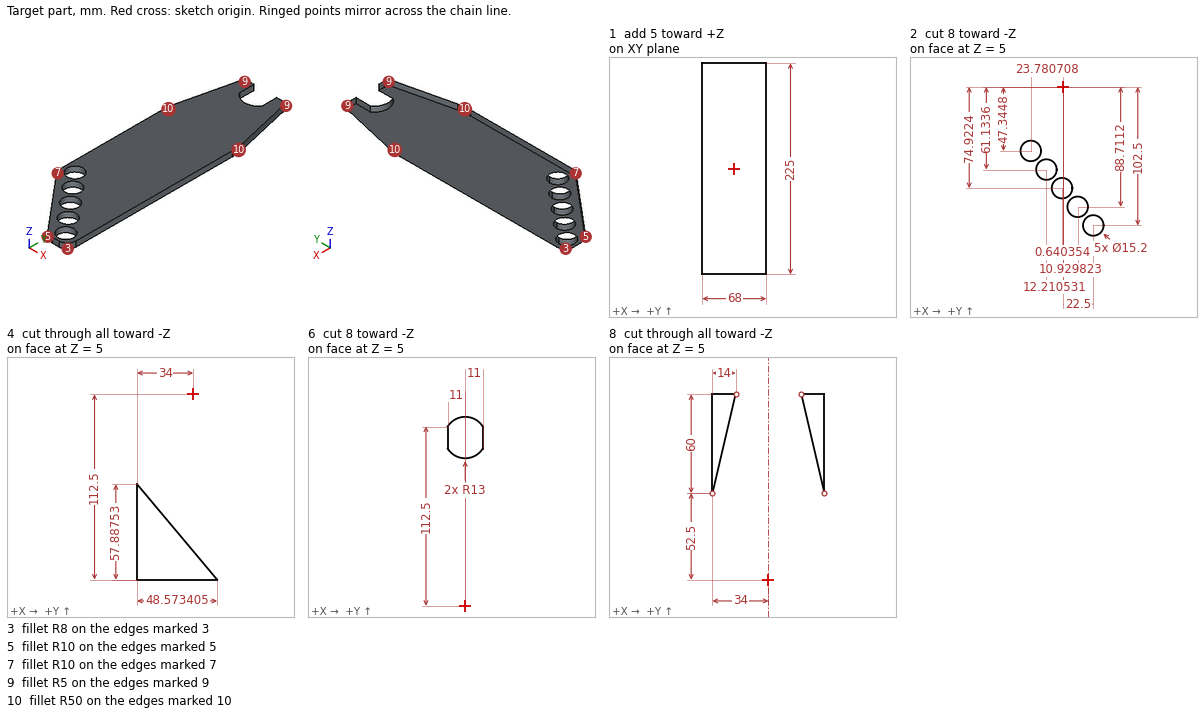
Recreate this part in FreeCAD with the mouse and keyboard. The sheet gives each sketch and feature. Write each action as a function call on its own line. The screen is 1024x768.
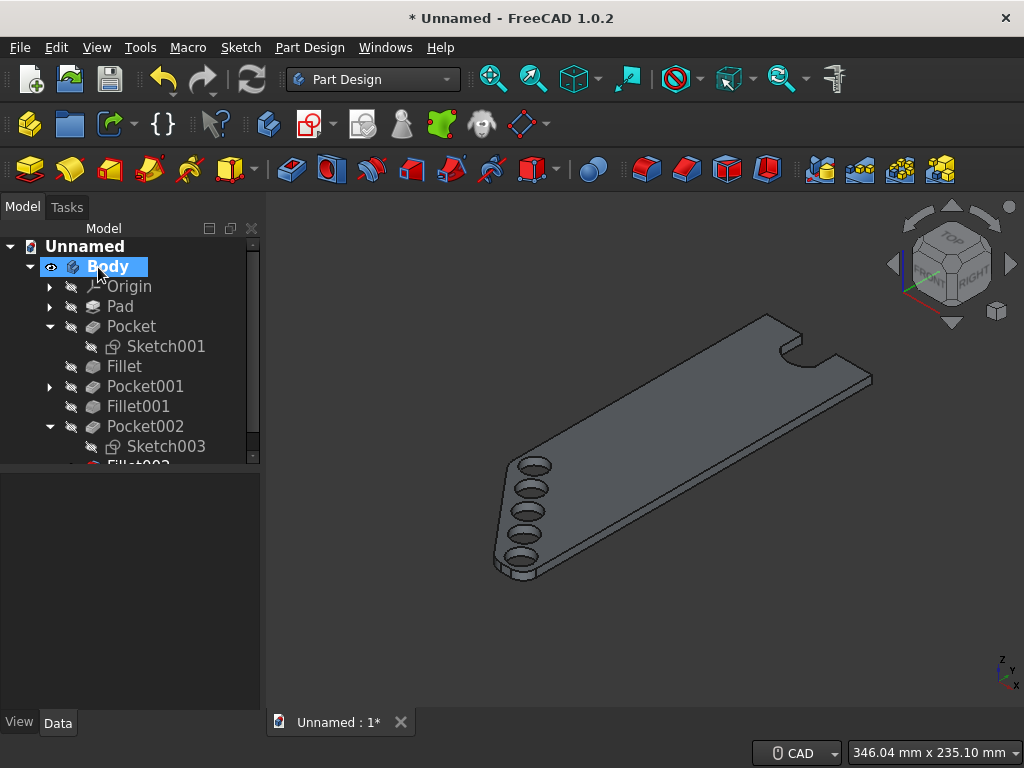
click(695, 415)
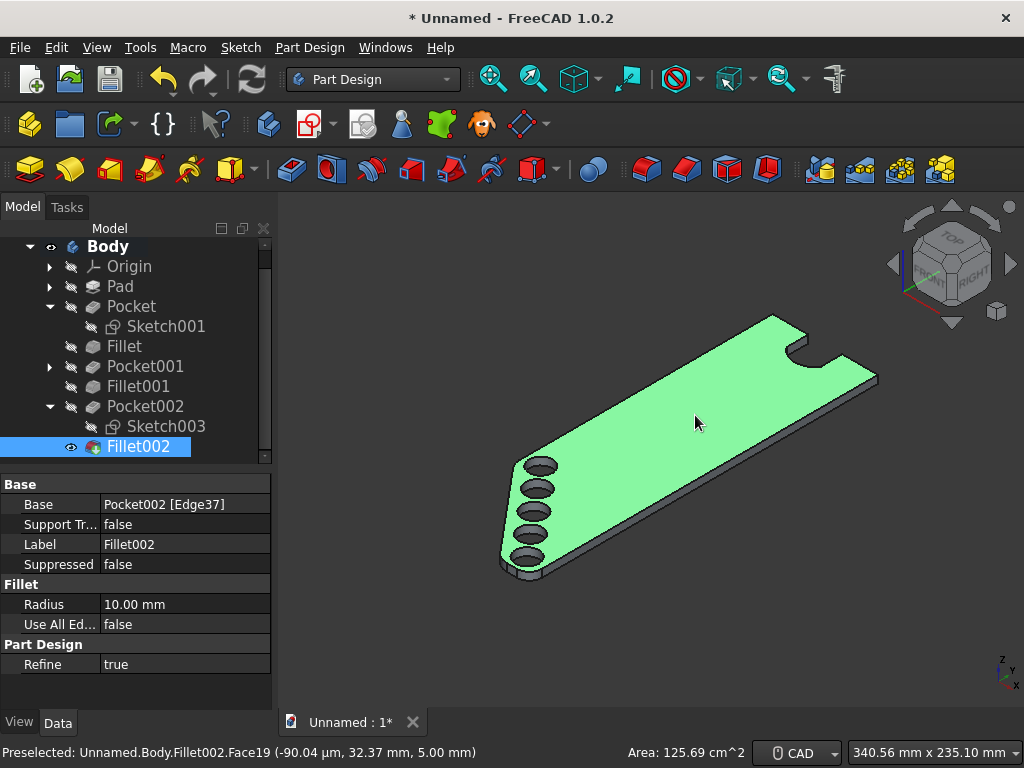
click(310, 124)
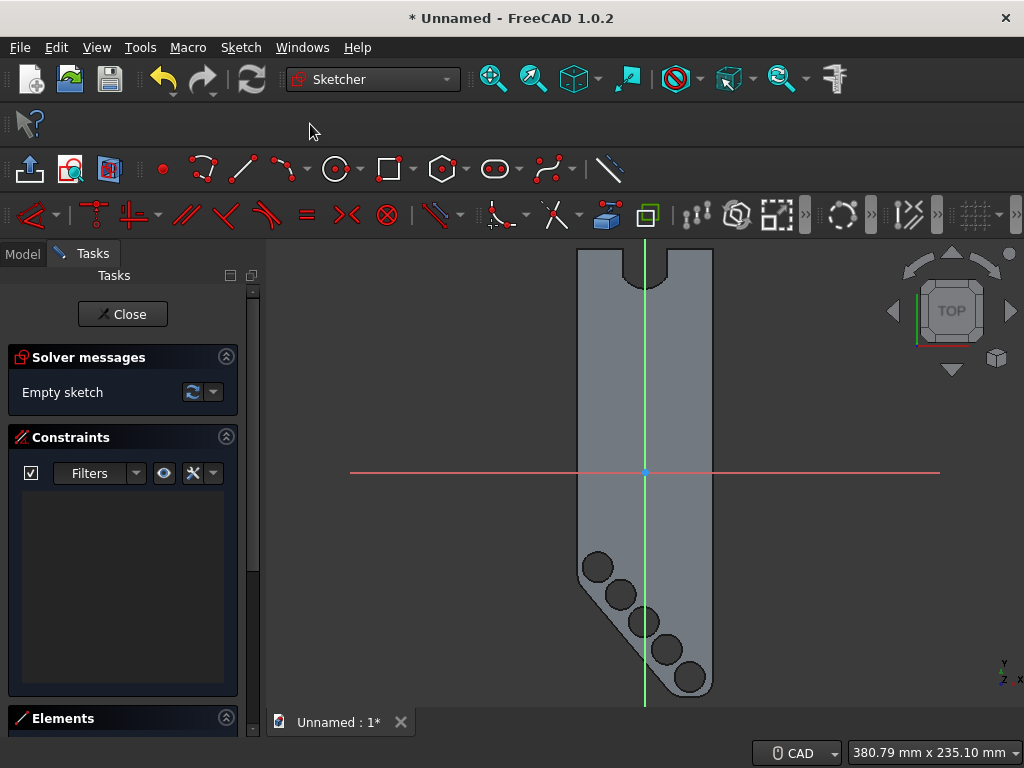
scroll(294, 679, down, 1)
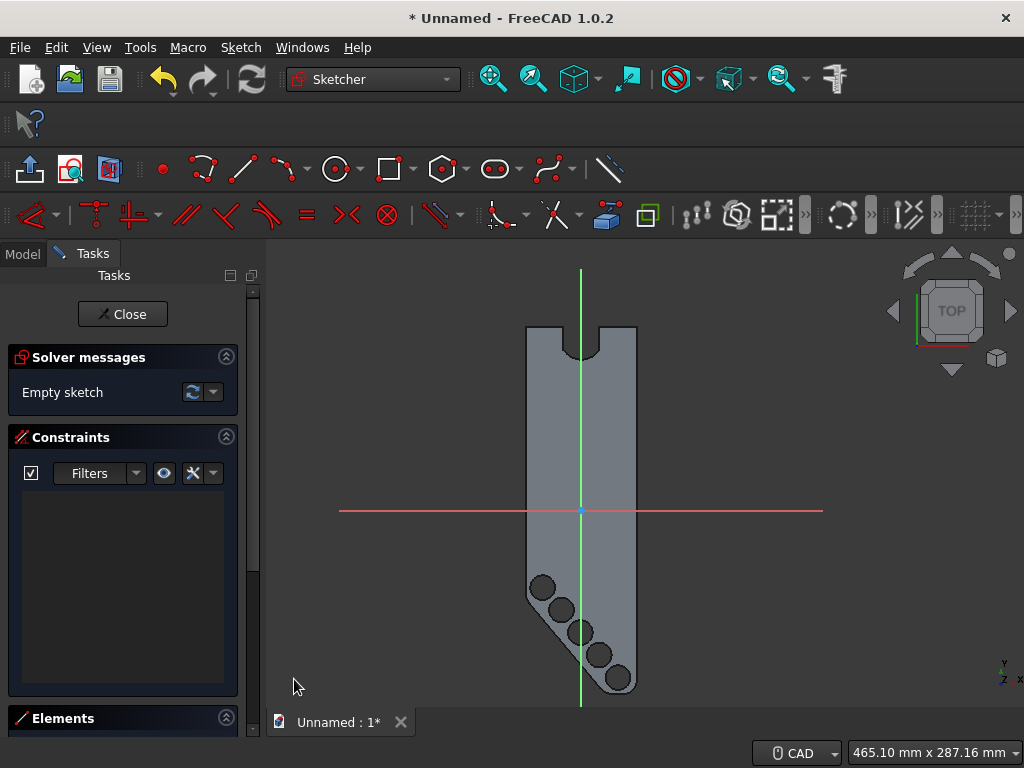
scroll(591, 309, up, 2)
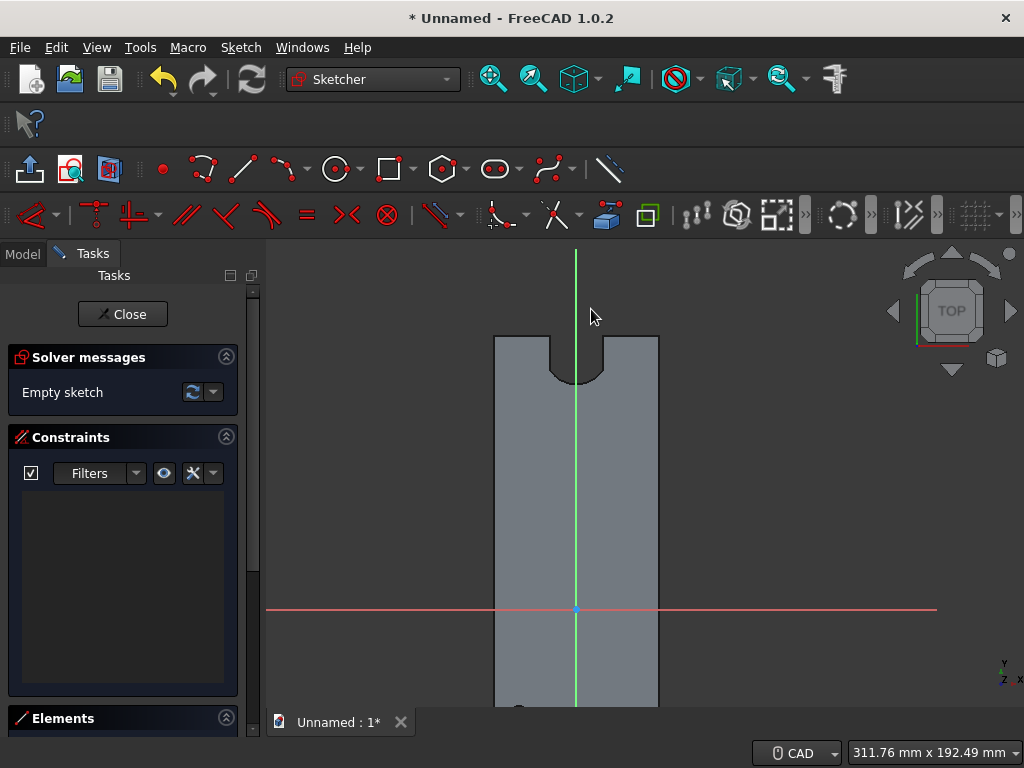
key(g)
key(m)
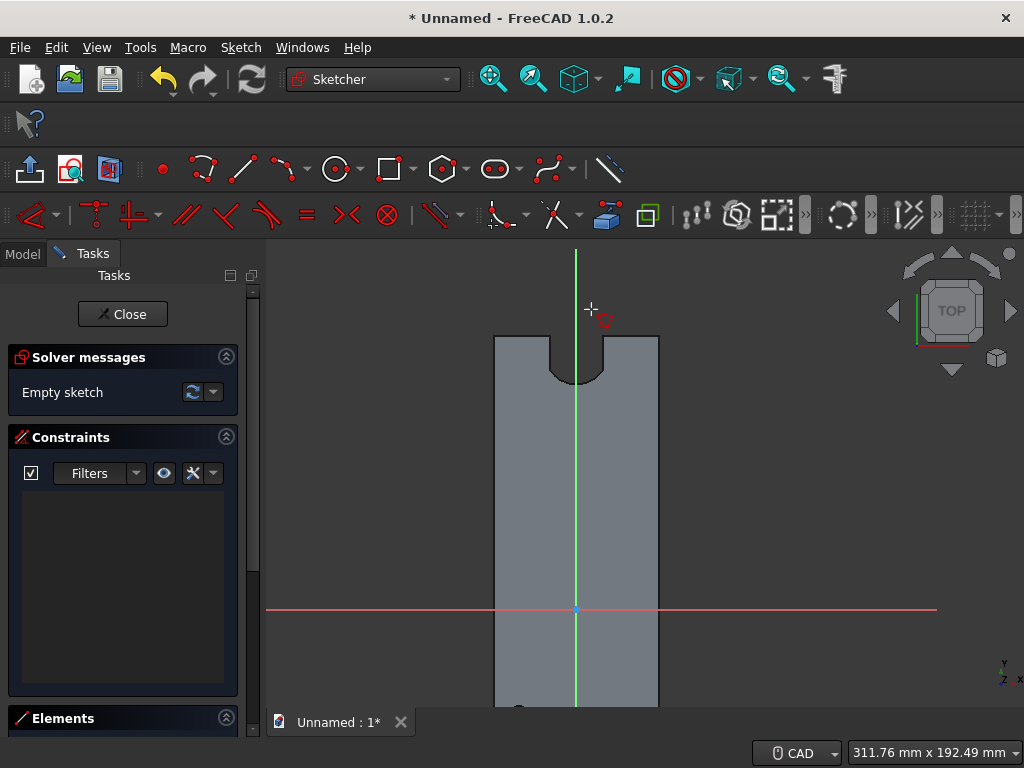
click(494, 482)
click(528, 336)
click(494, 336)
click(494, 483)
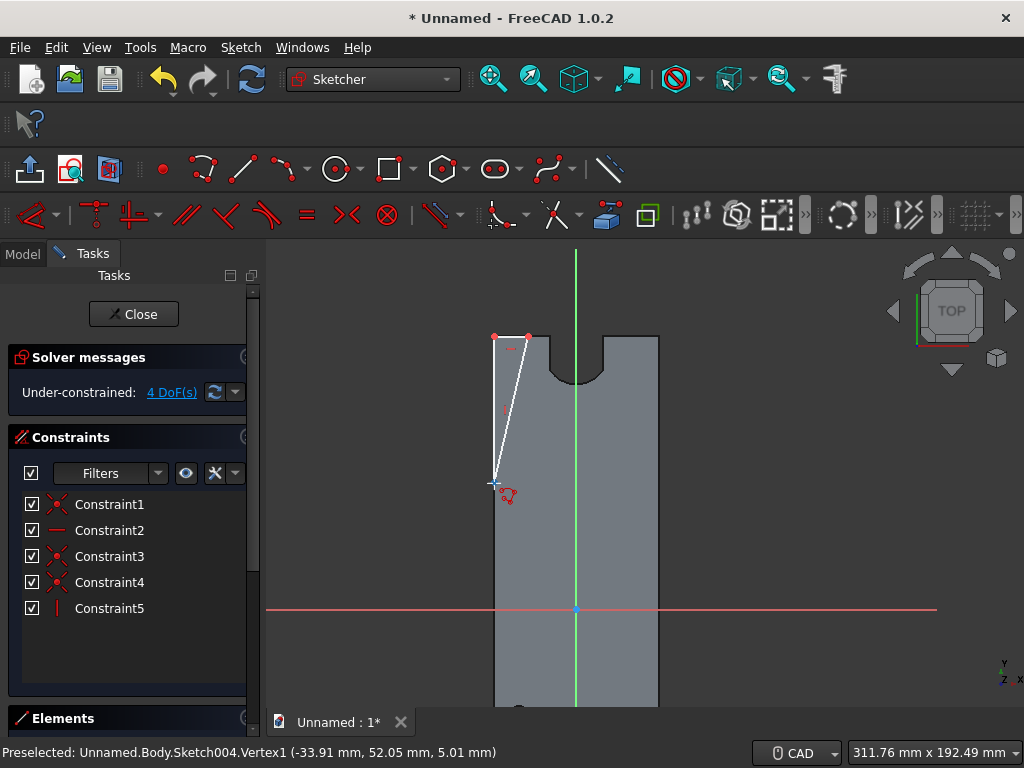
click(659, 482)
click(659, 336)
click(625, 336)
click(659, 483)
key(Escape)
key(Escape)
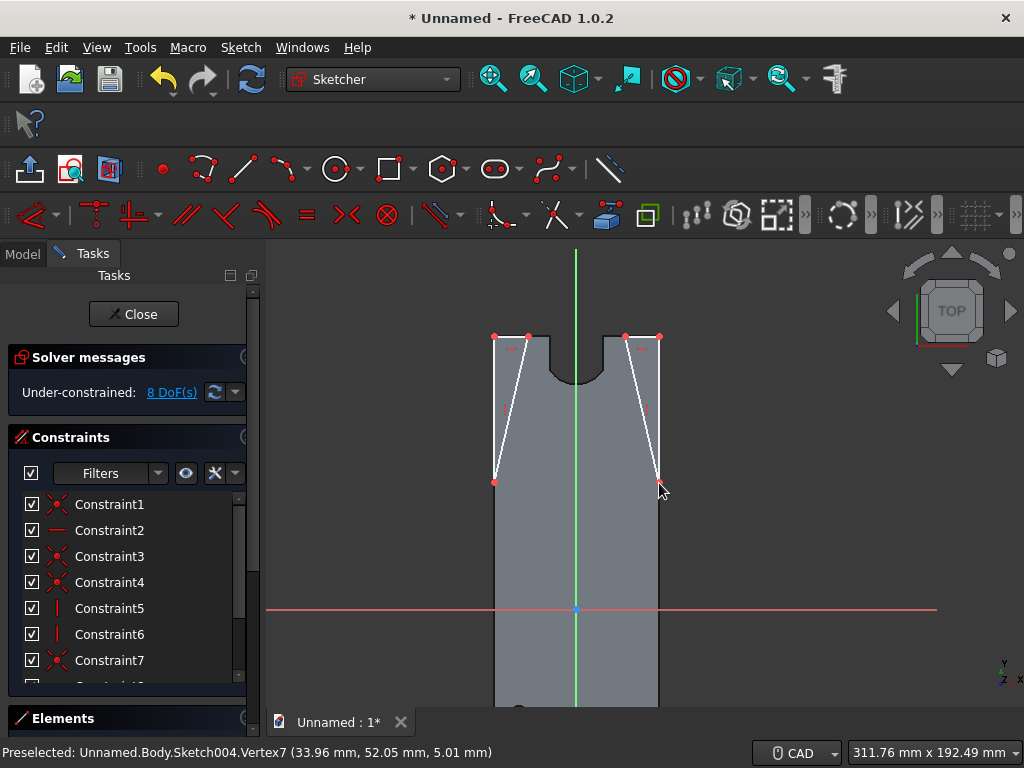
click(494, 483)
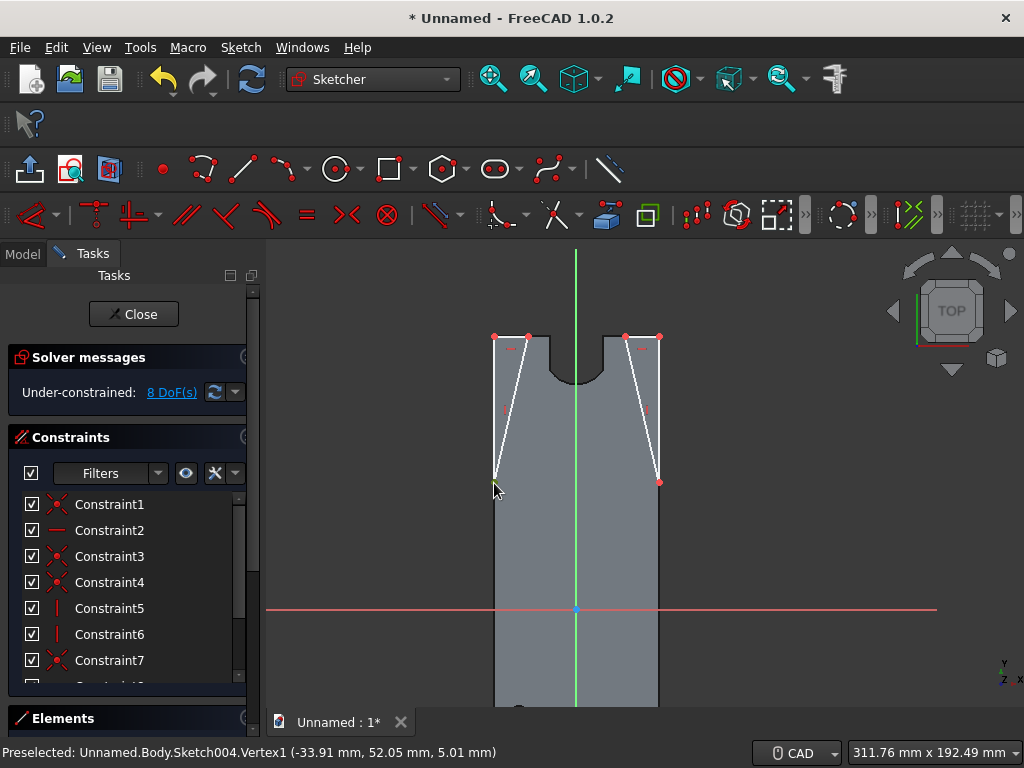
click(659, 483)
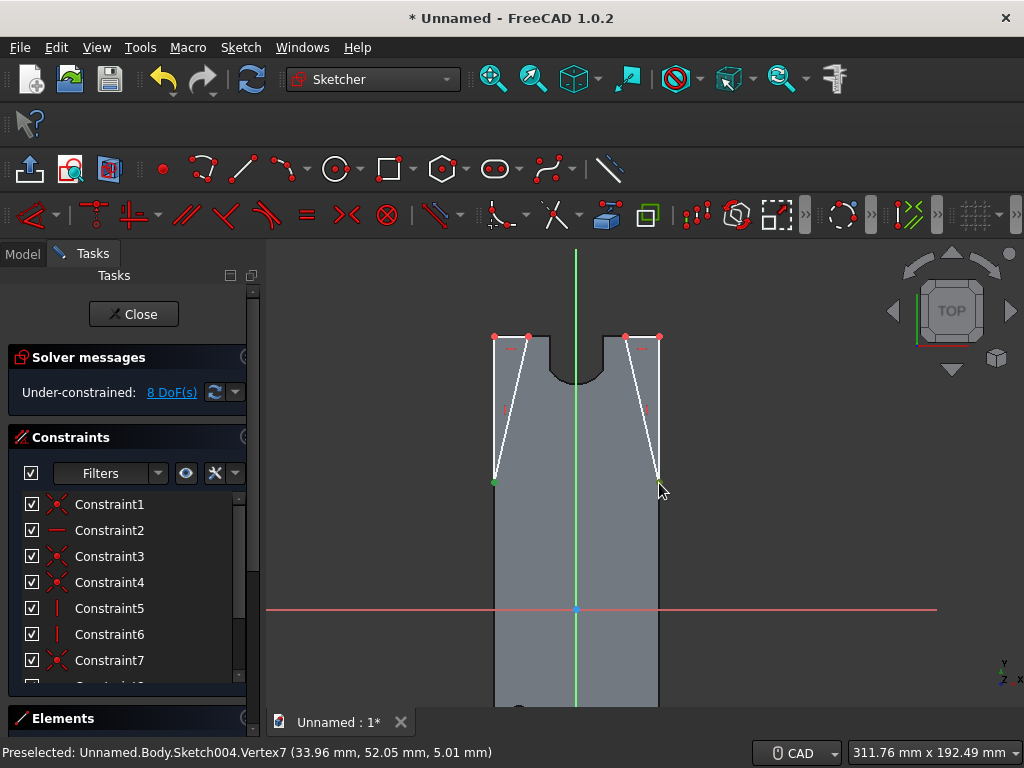
click(576, 650)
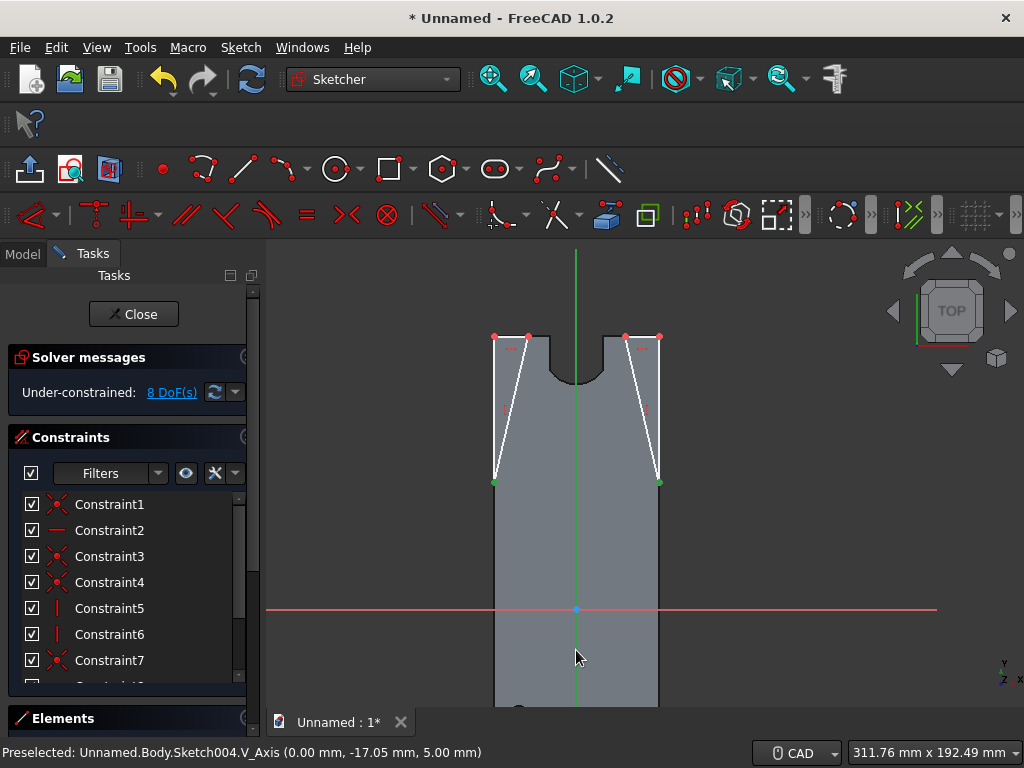
click(348, 216)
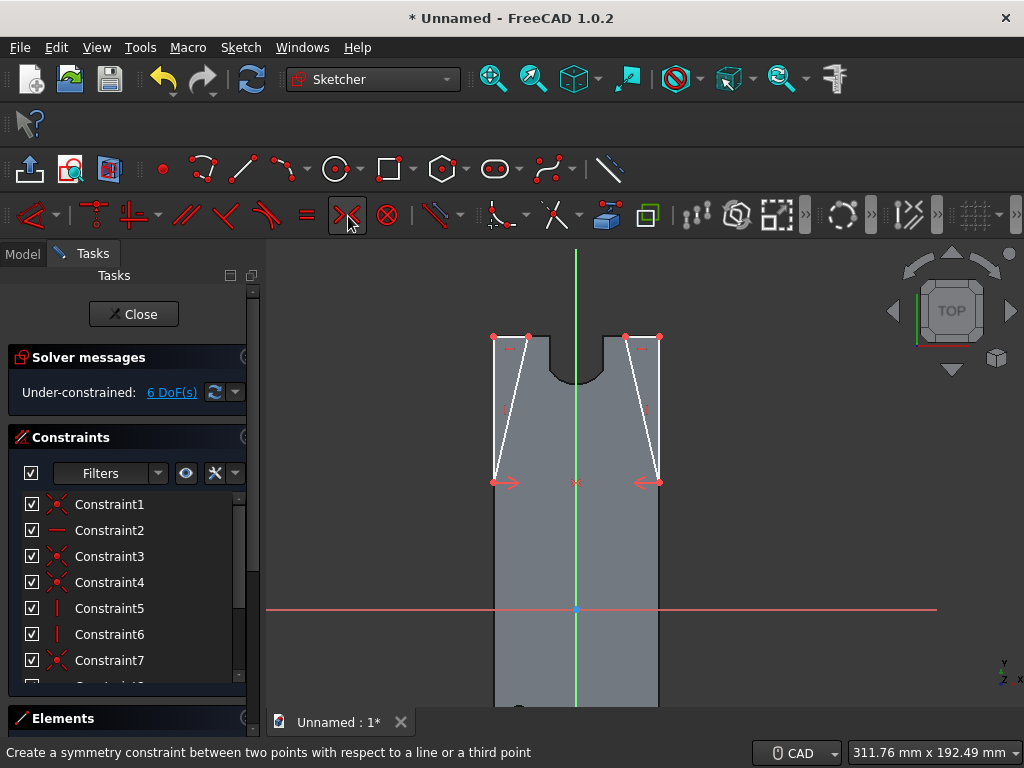
click(528, 337)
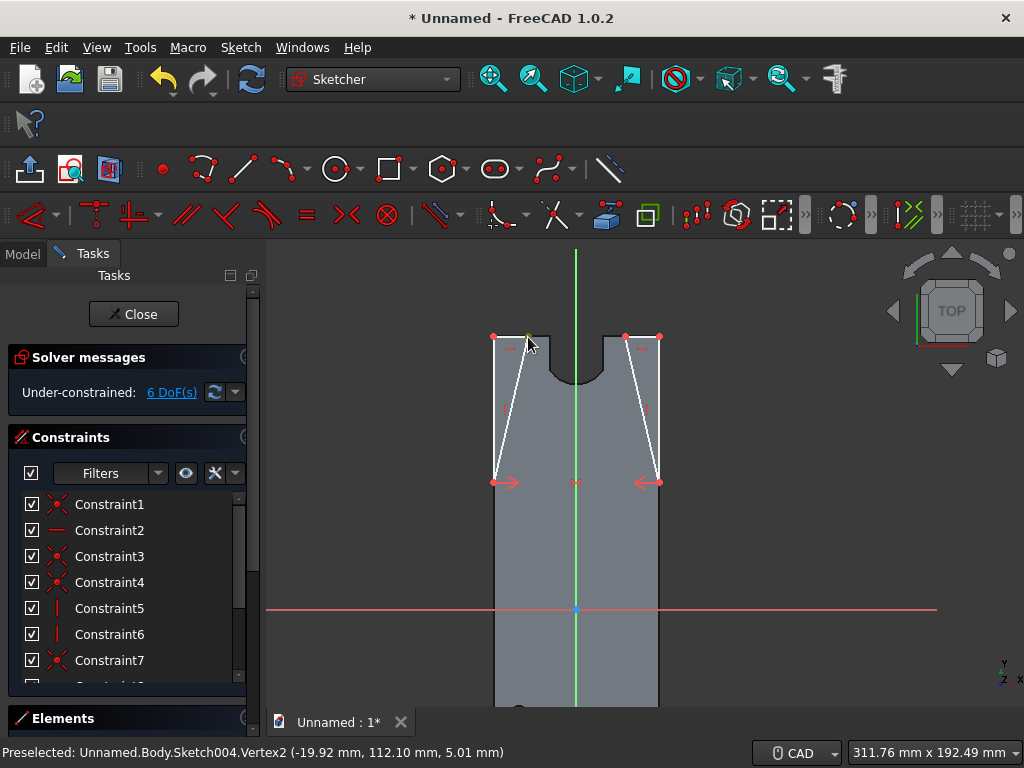
click(625, 337)